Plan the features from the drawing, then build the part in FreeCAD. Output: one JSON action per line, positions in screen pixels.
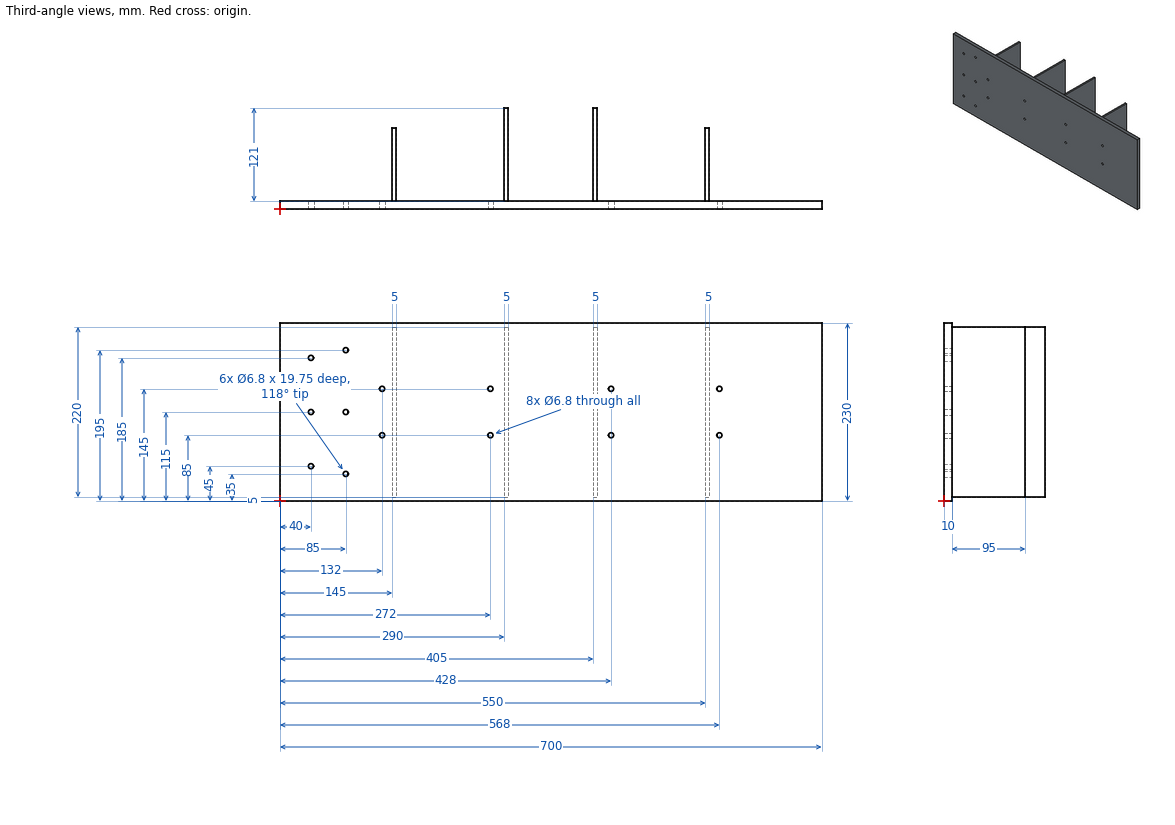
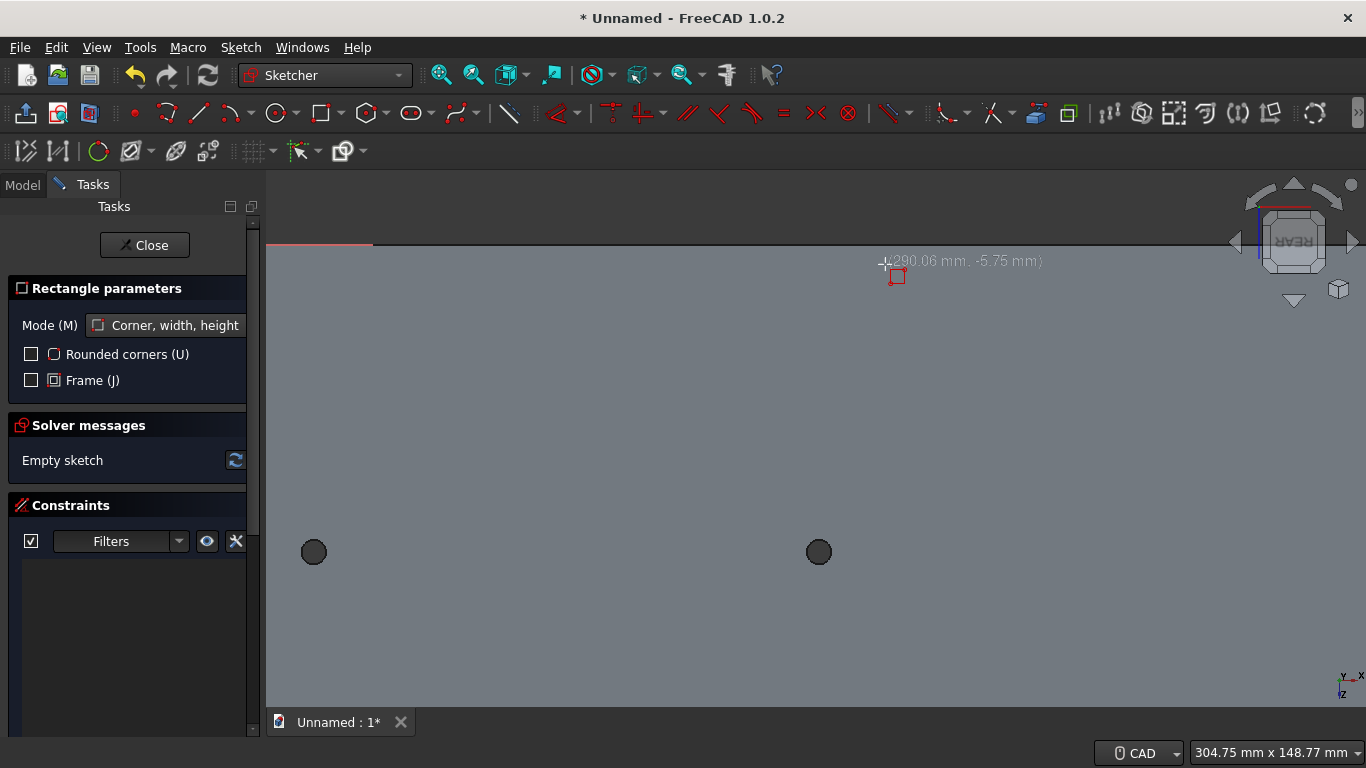
{"action": "left_click", "coordinate": [884, 263]}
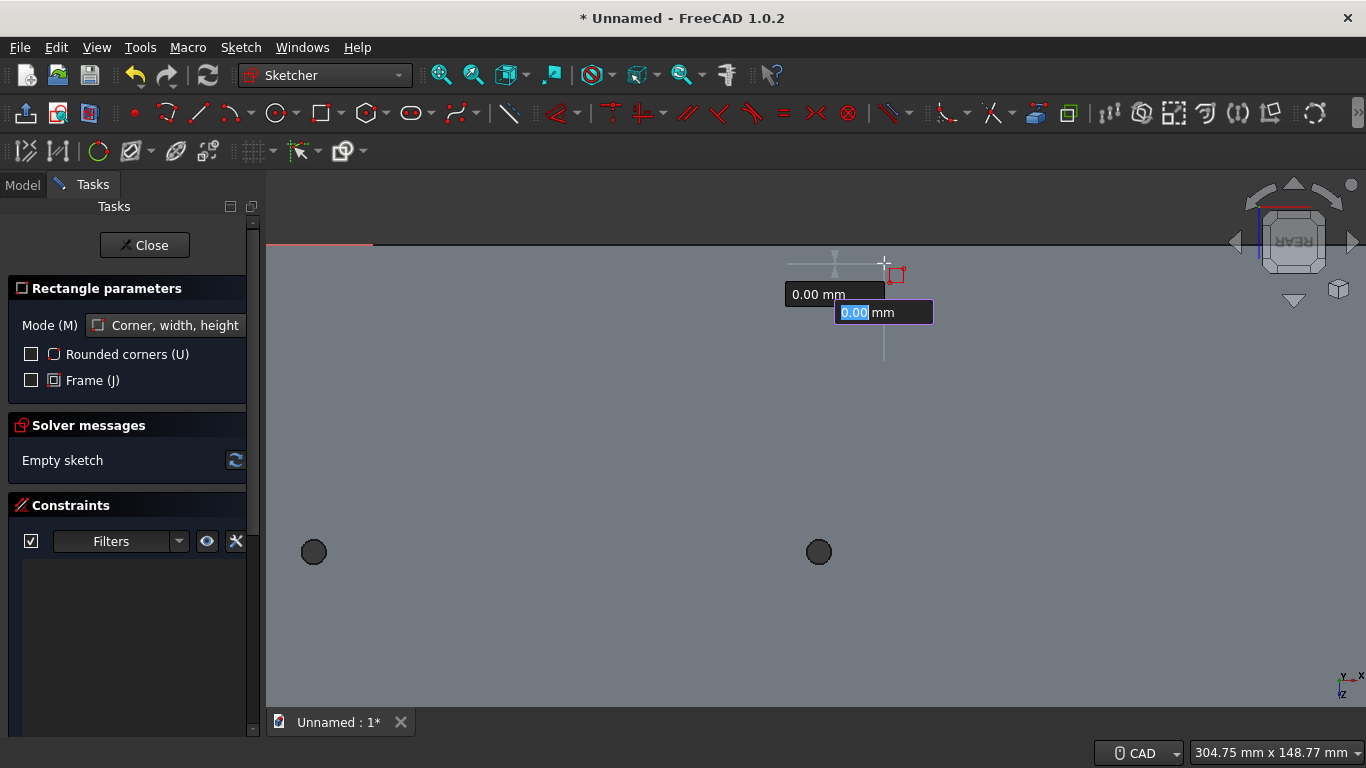
{"action": "scroll", "coordinate": [886, 265], "scroll_direction": "down", "scroll_amount": 4}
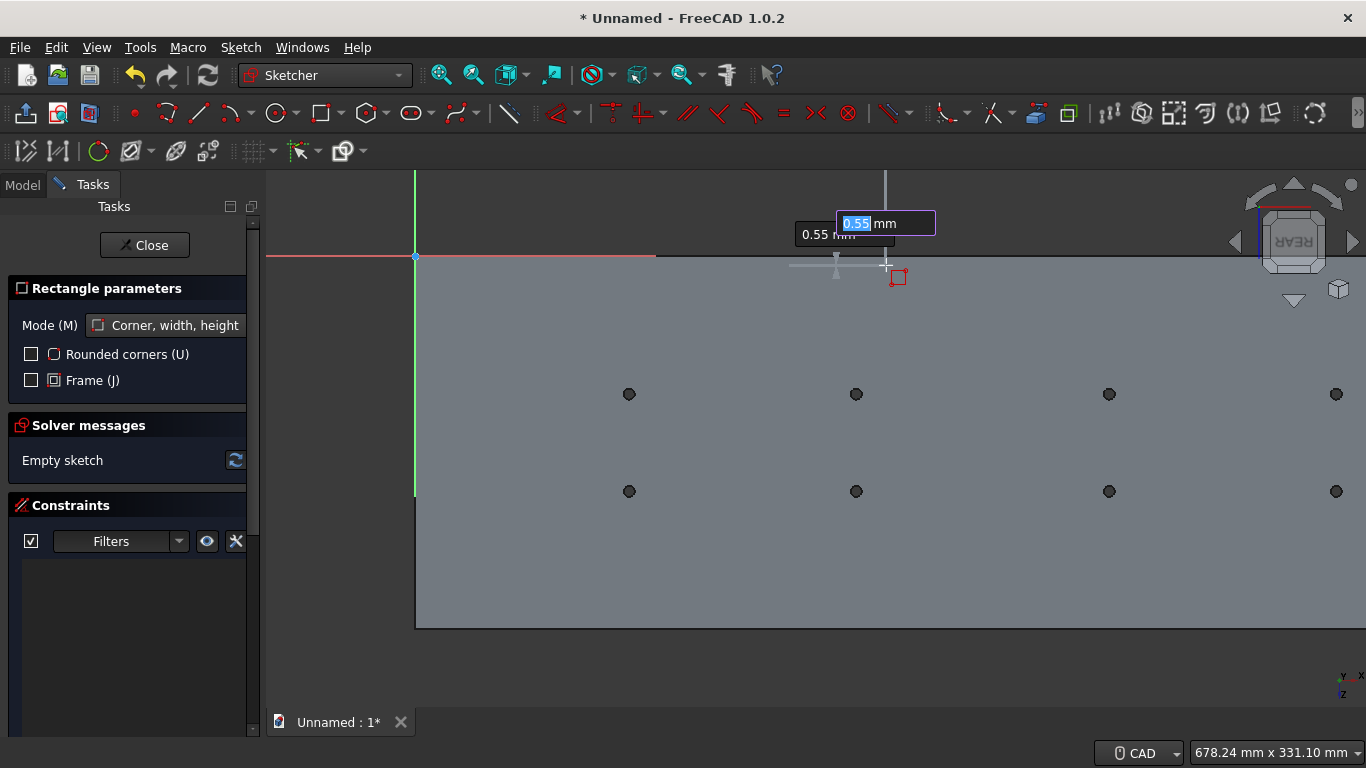
{"action": "left_click", "coordinate": [894, 621]}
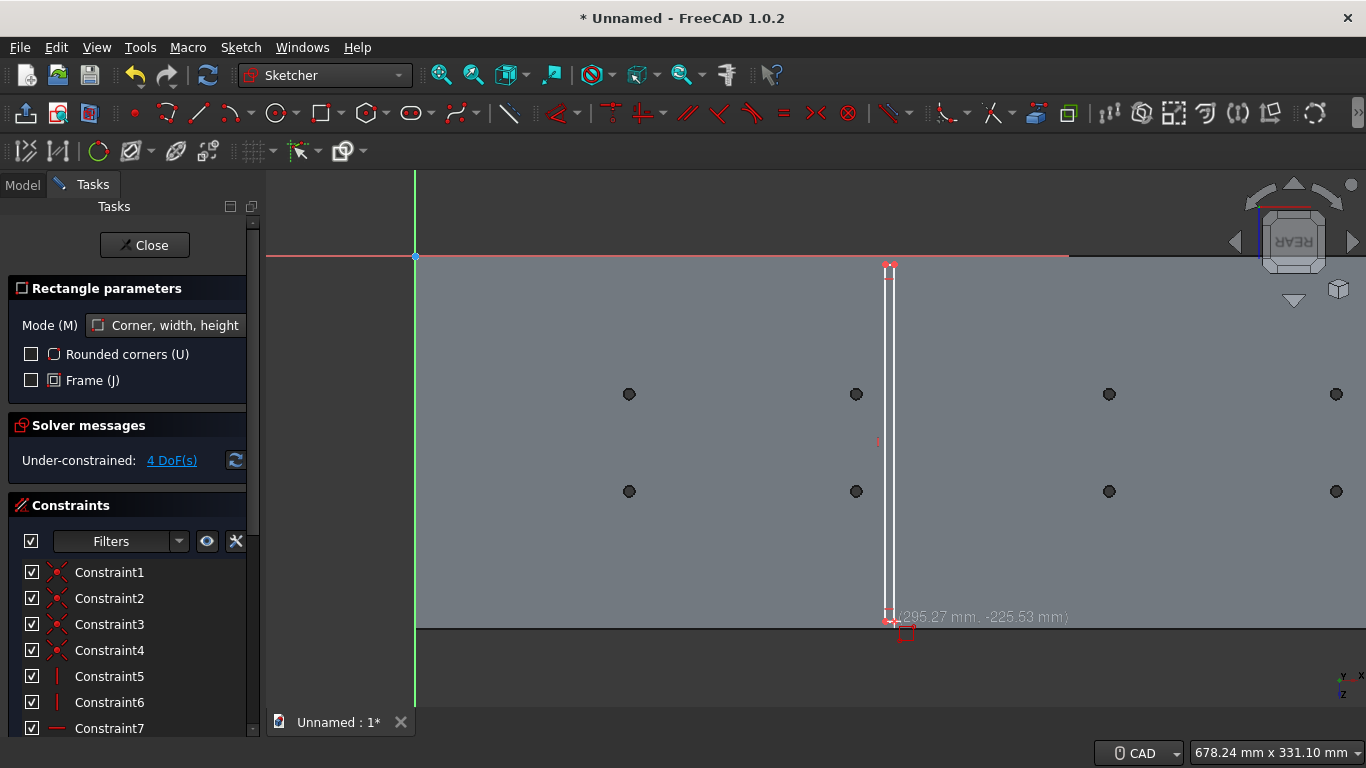
{"action": "scroll", "coordinate": [1072, 264], "scroll_direction": "up", "scroll_amount": 4}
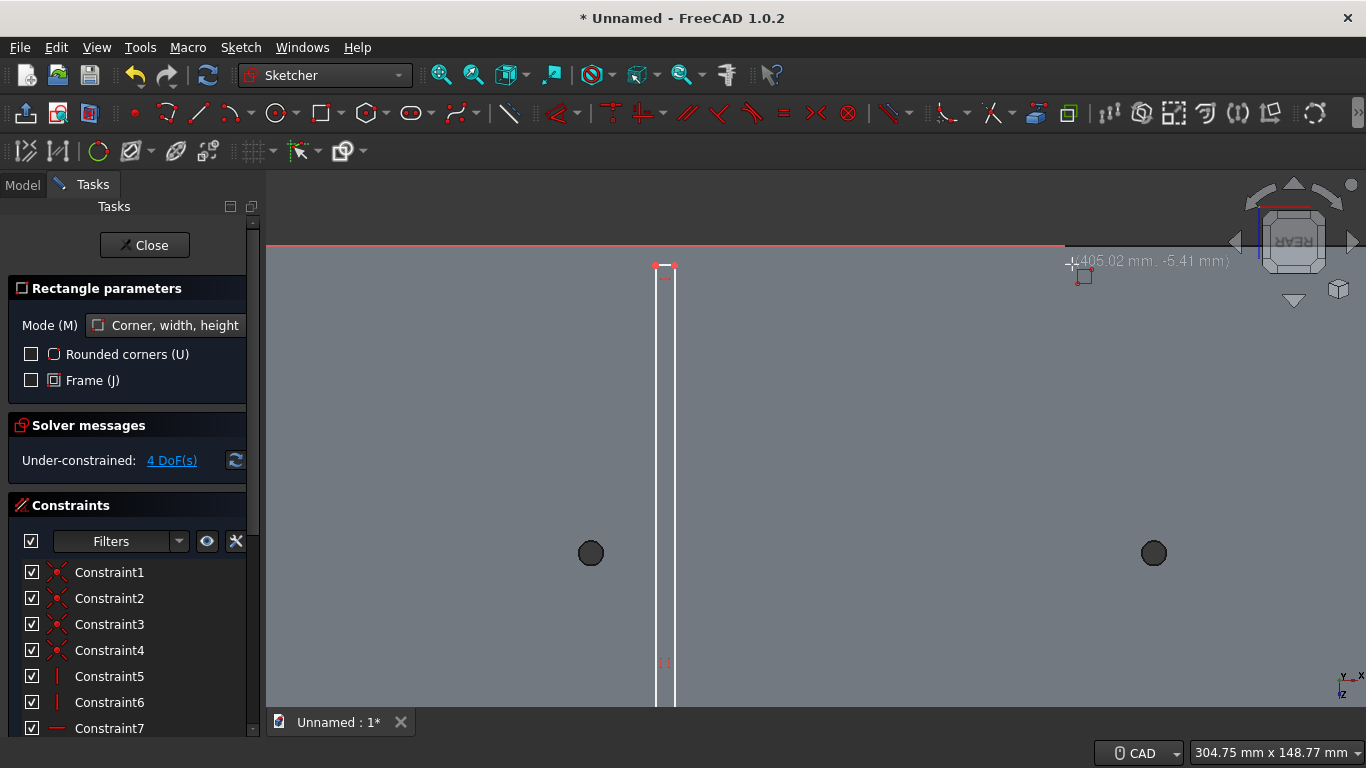
{"action": "left_click", "coordinate": [1071, 265]}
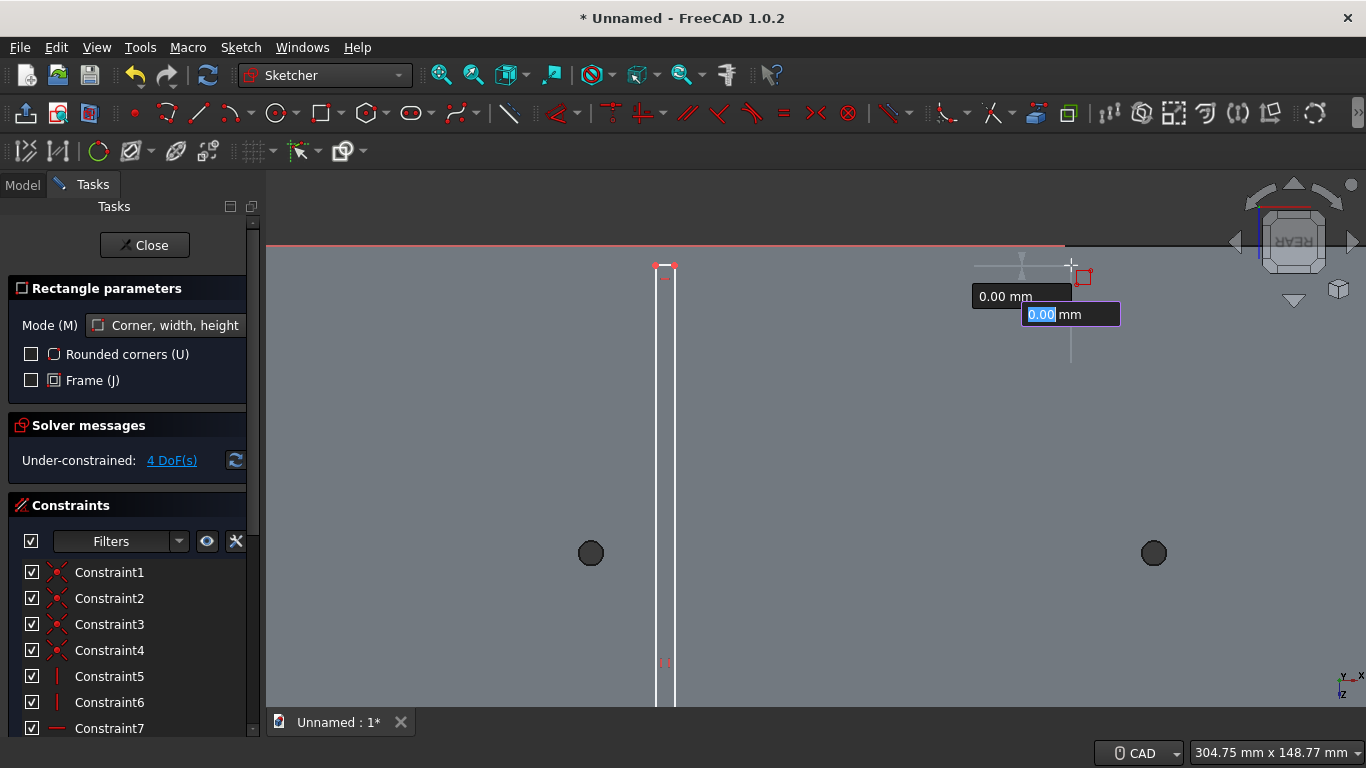
{"action": "scroll", "coordinate": [1073, 264], "scroll_direction": "down", "scroll_amount": 4}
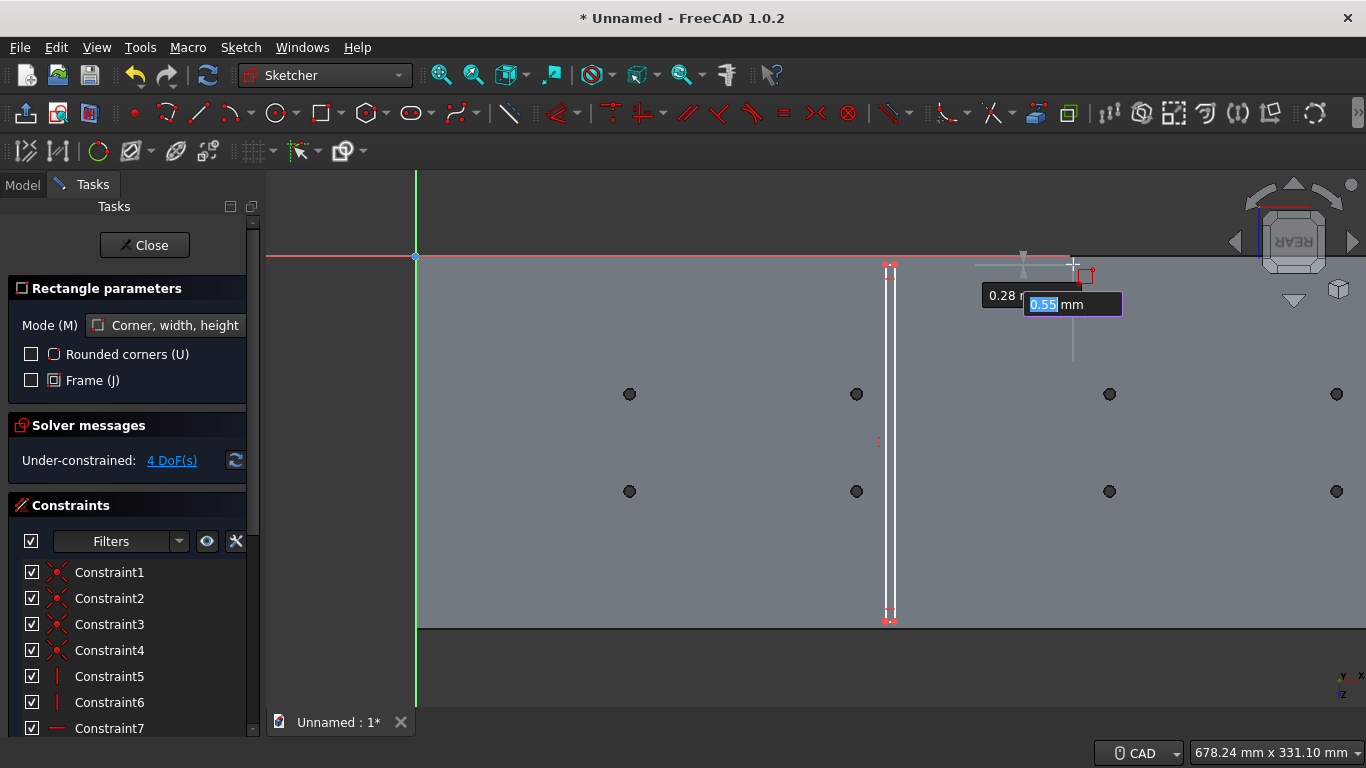
{"action": "left_click", "coordinate": [1081, 621]}
{"action": "key", "text": "Escape"}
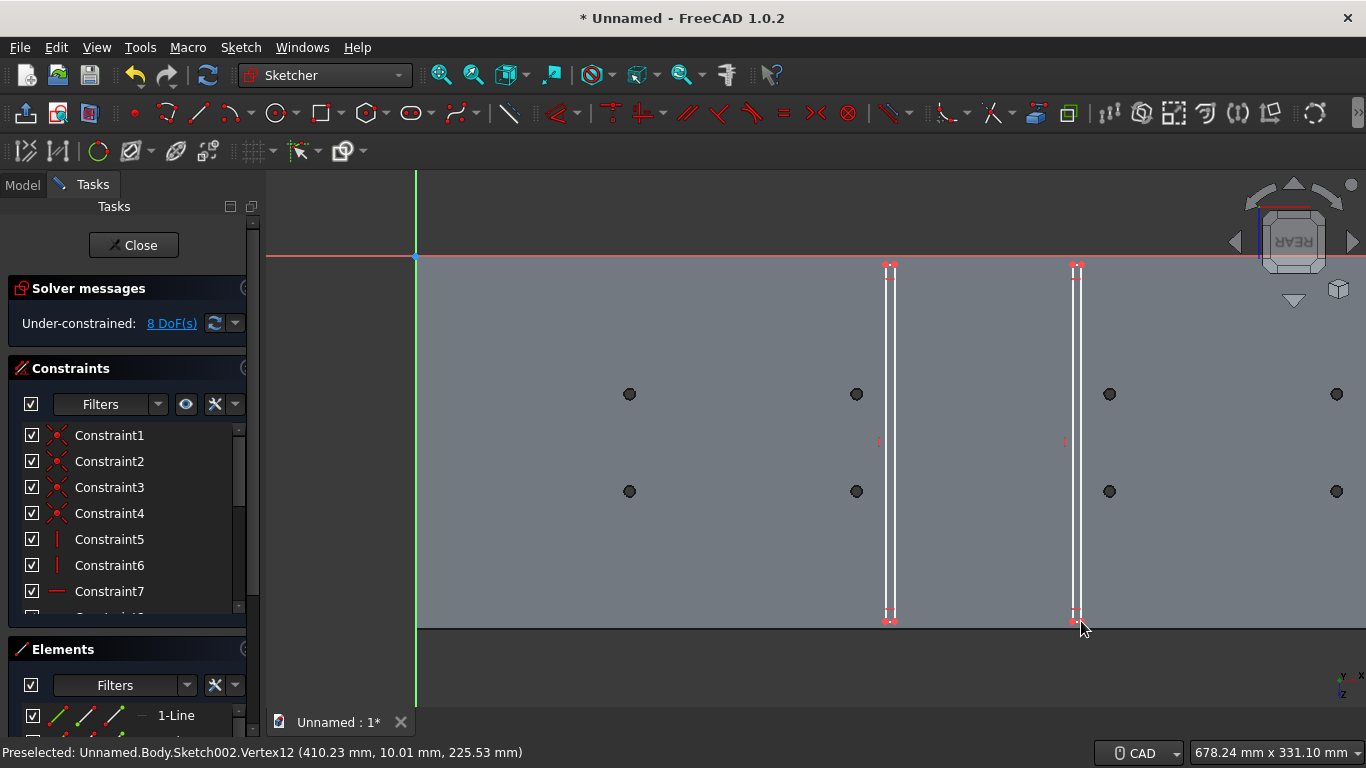
{"action": "key", "text": "d"}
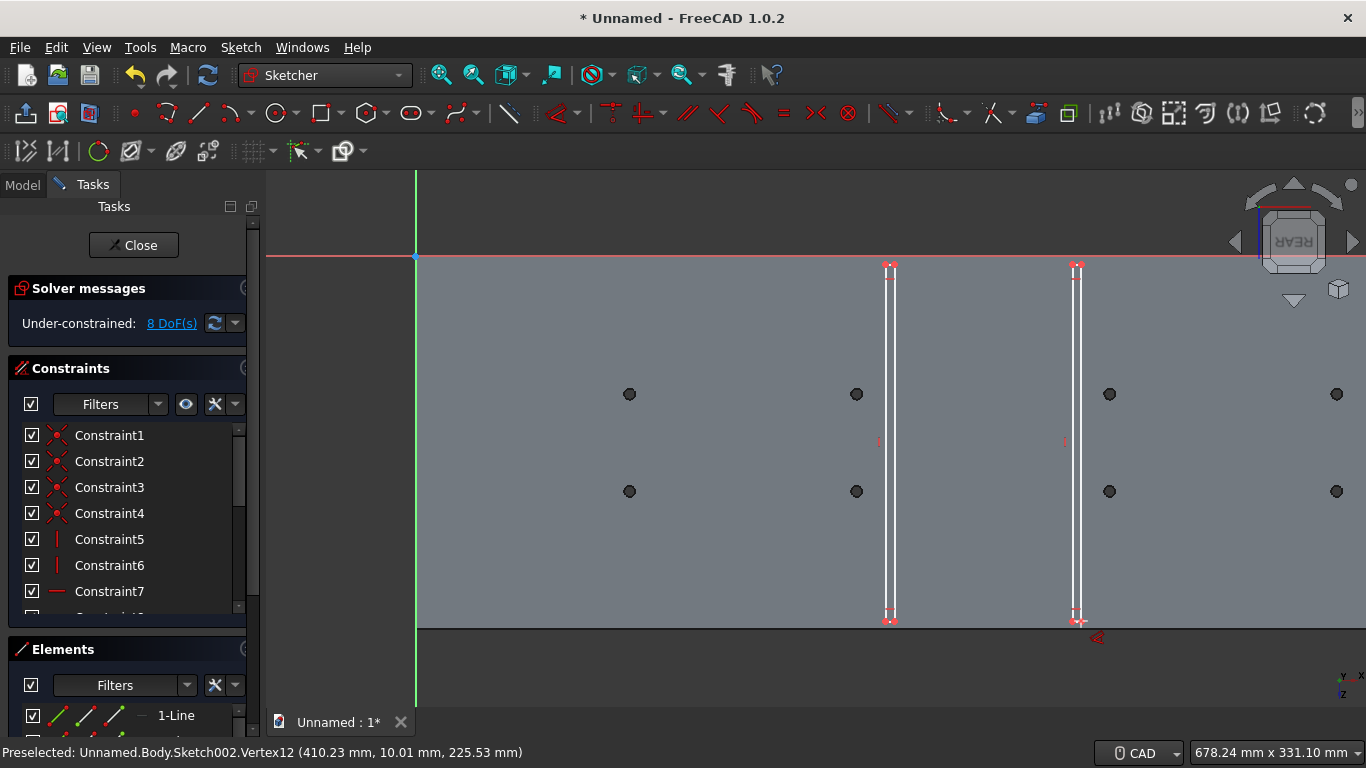
{"action": "scroll", "coordinate": [890, 622], "scroll_direction": "up", "scroll_amount": 8}